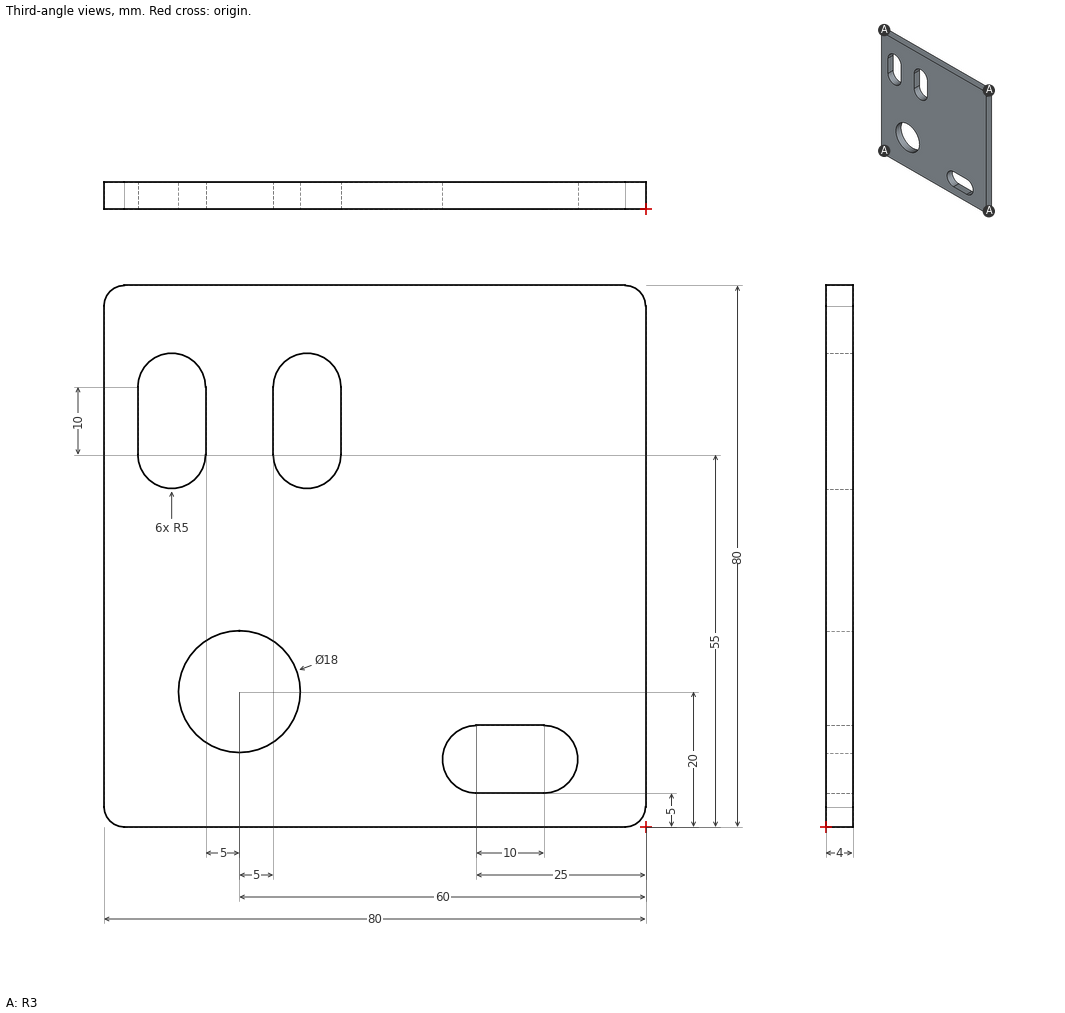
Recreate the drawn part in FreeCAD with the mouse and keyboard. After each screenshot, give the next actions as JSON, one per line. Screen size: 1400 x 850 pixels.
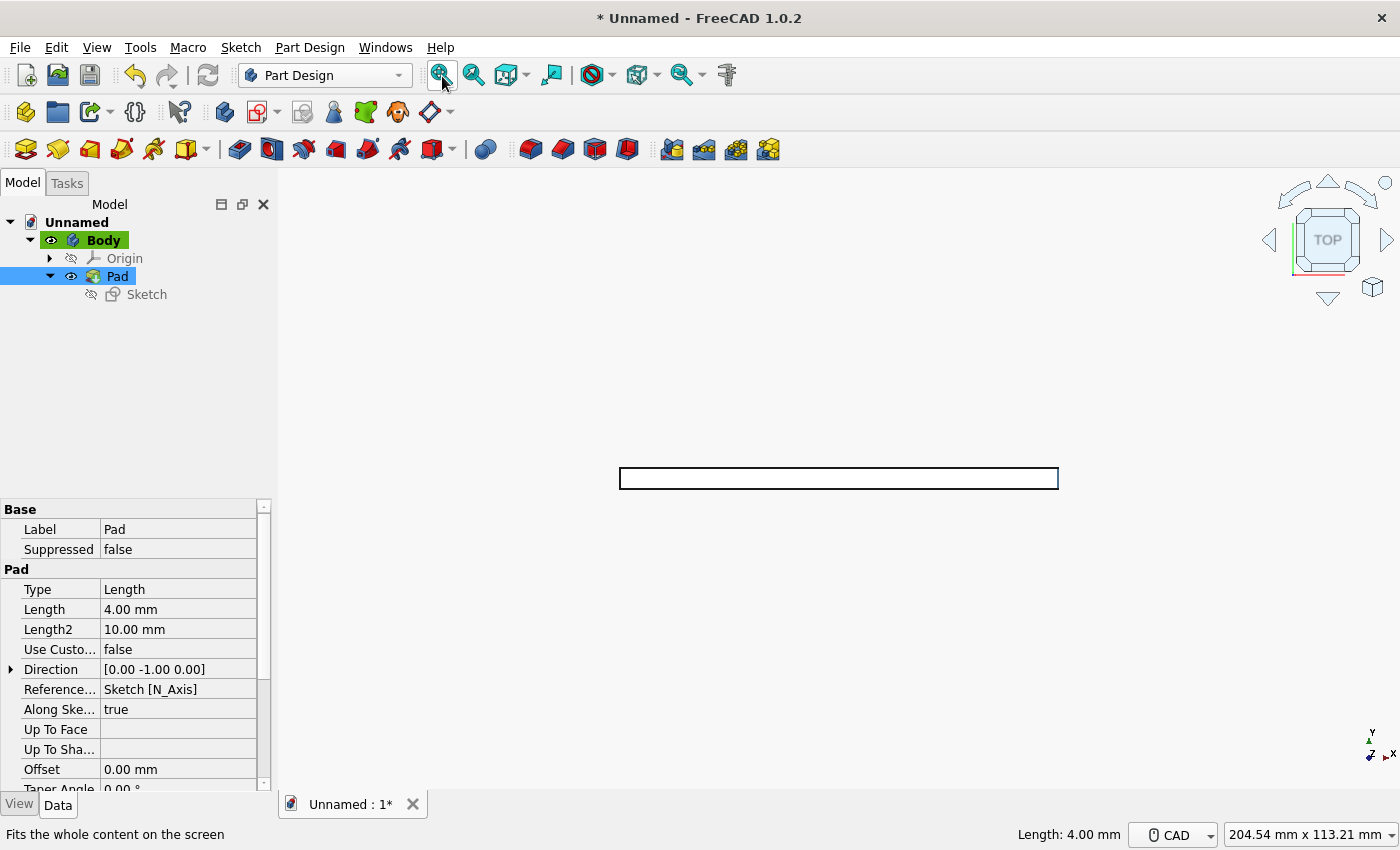
{"action": "left_click", "coordinate": [442, 76]}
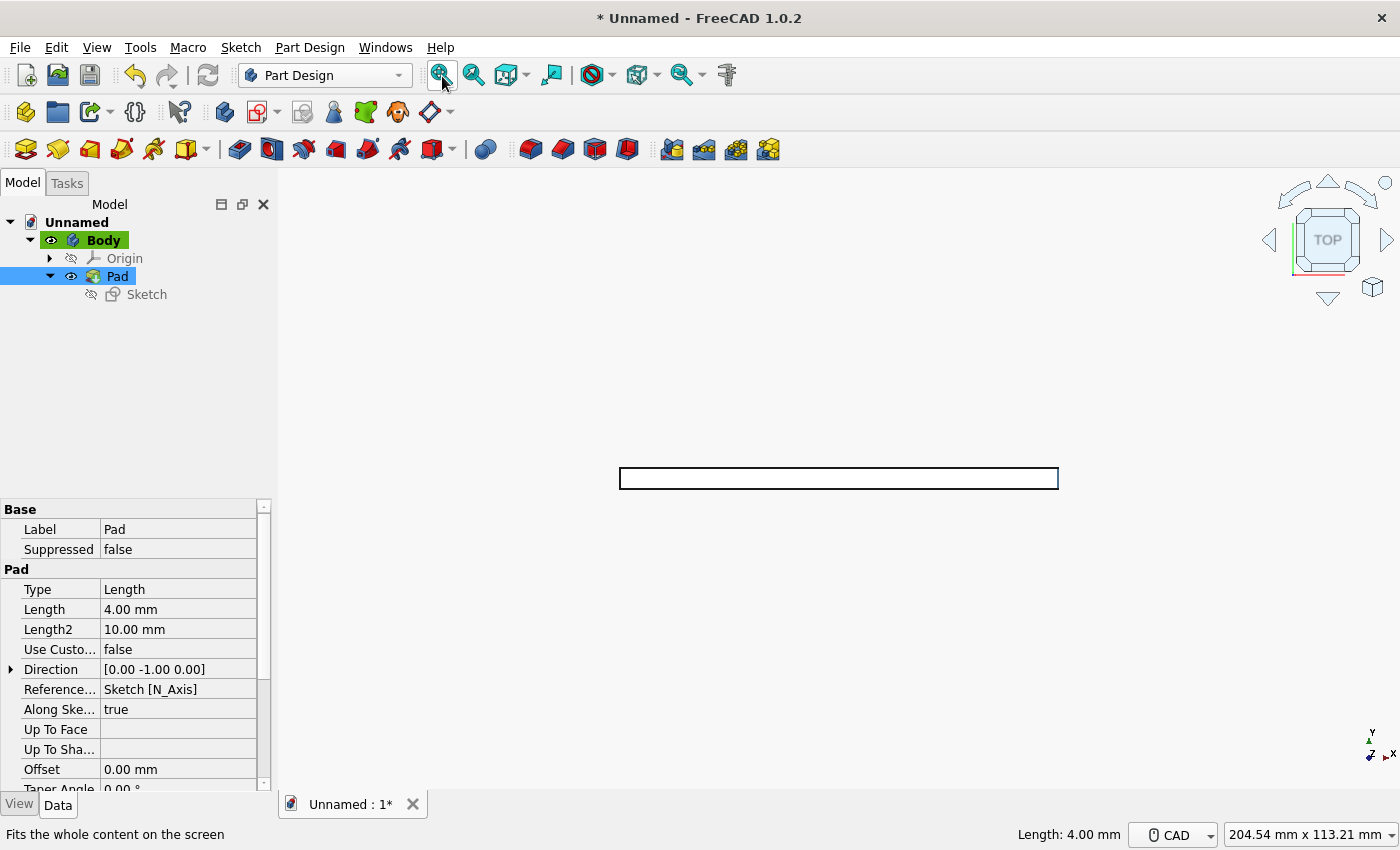
{"action": "left_click", "coordinate": [620, 477], "text": "ctrl"}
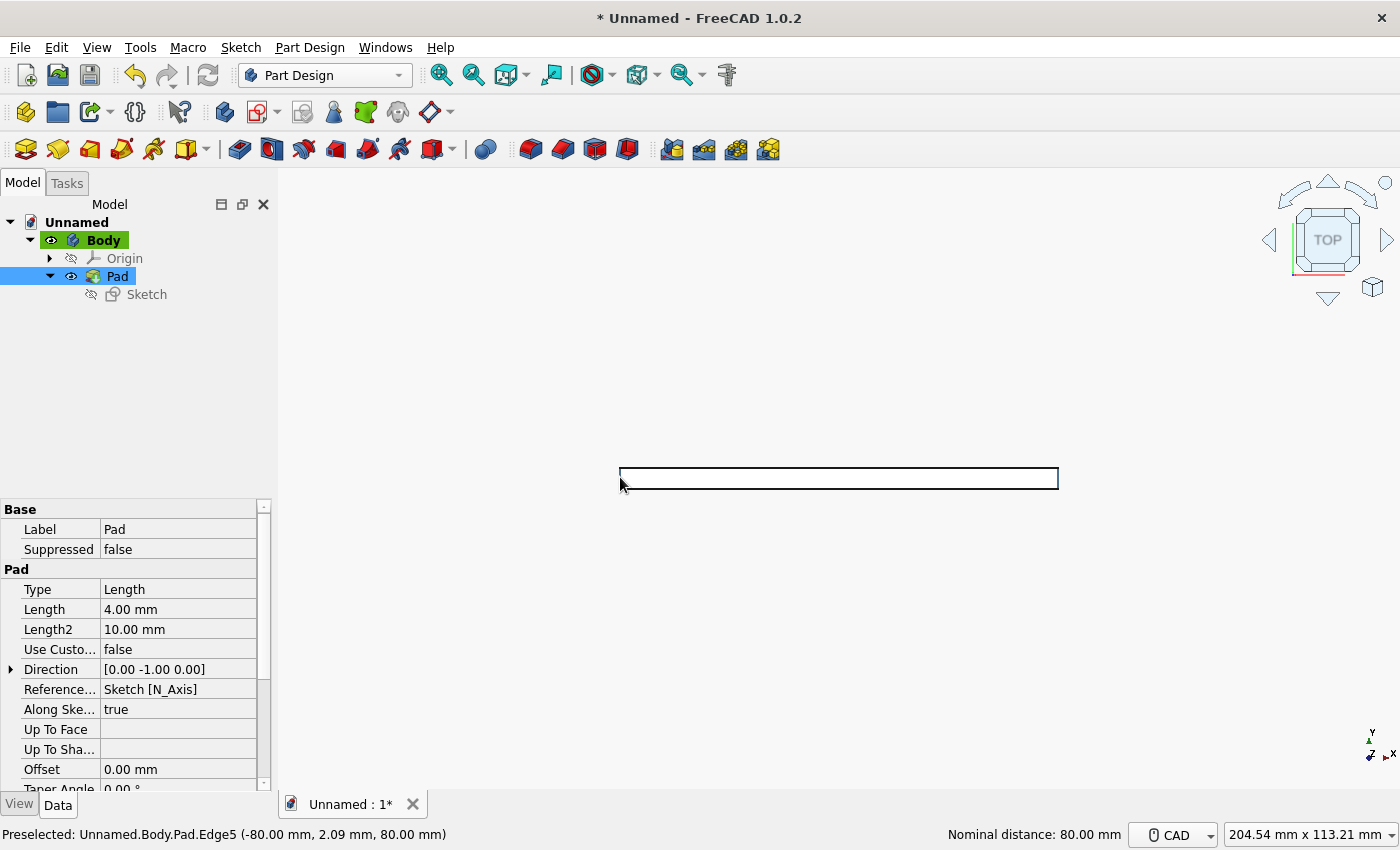
{"action": "scroll", "coordinate": [620, 477], "scroll_direction": "up", "scroll_amount": 4}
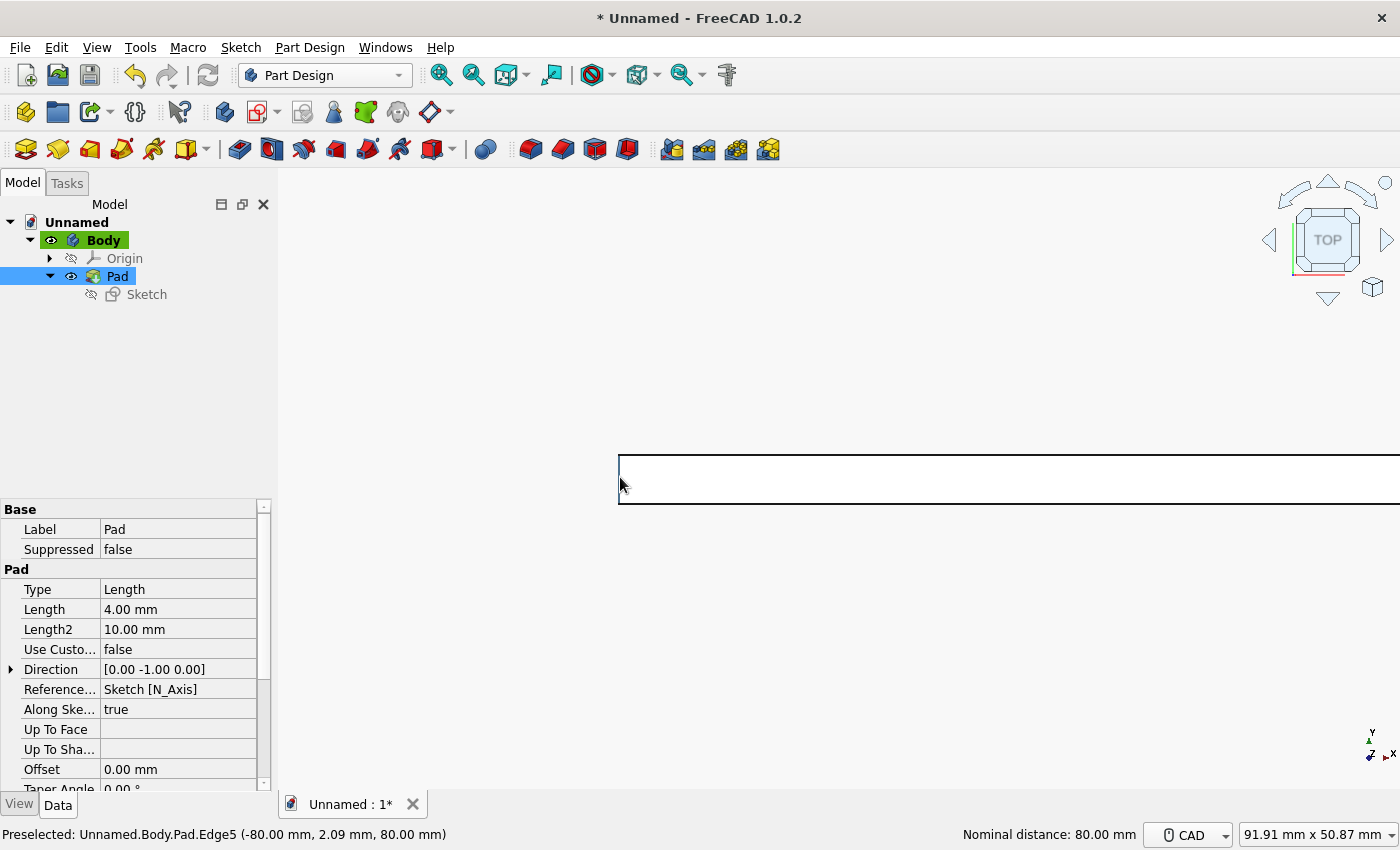
{"action": "left_click", "coordinate": [442, 76]}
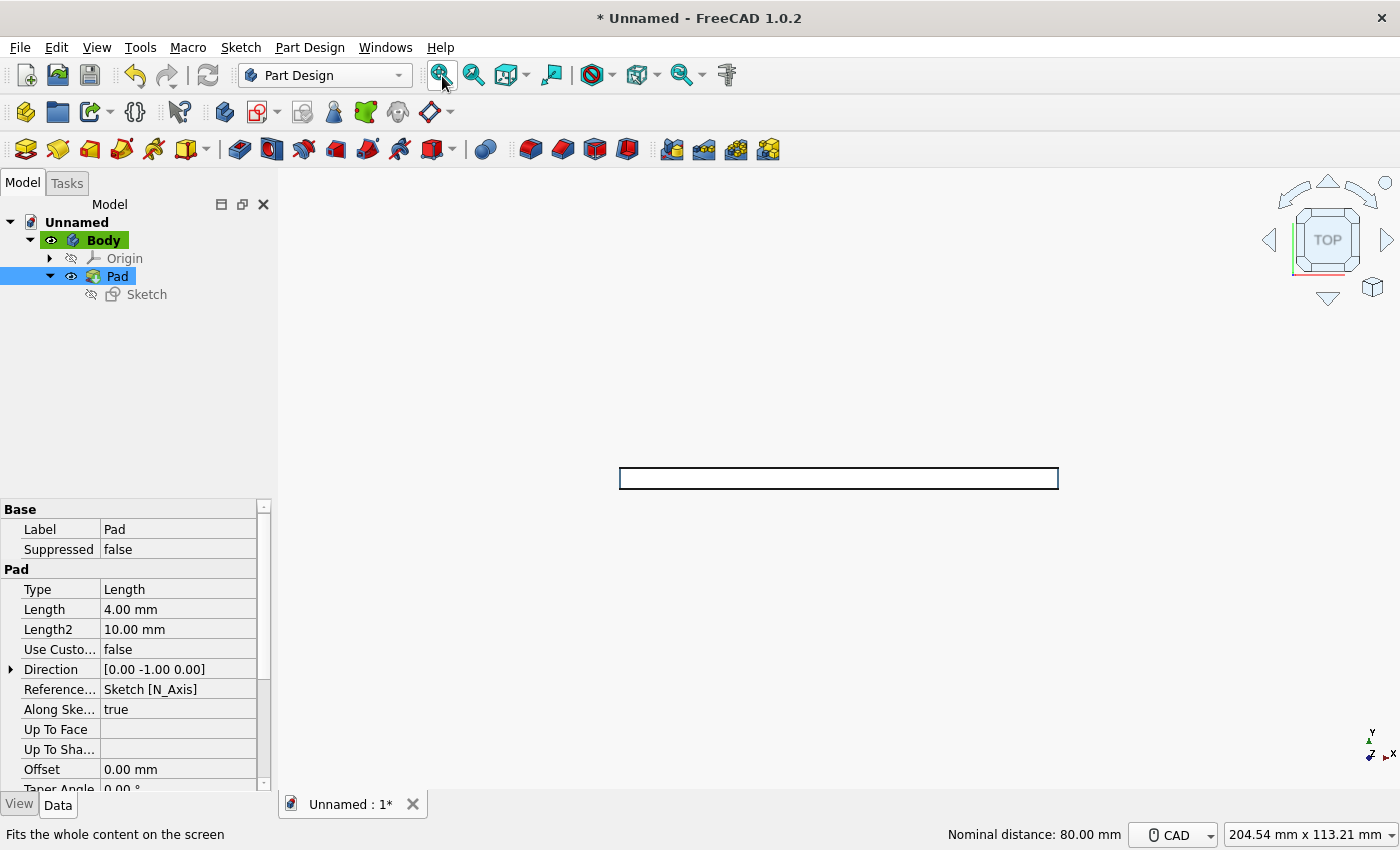
{"action": "key", "text": "1"}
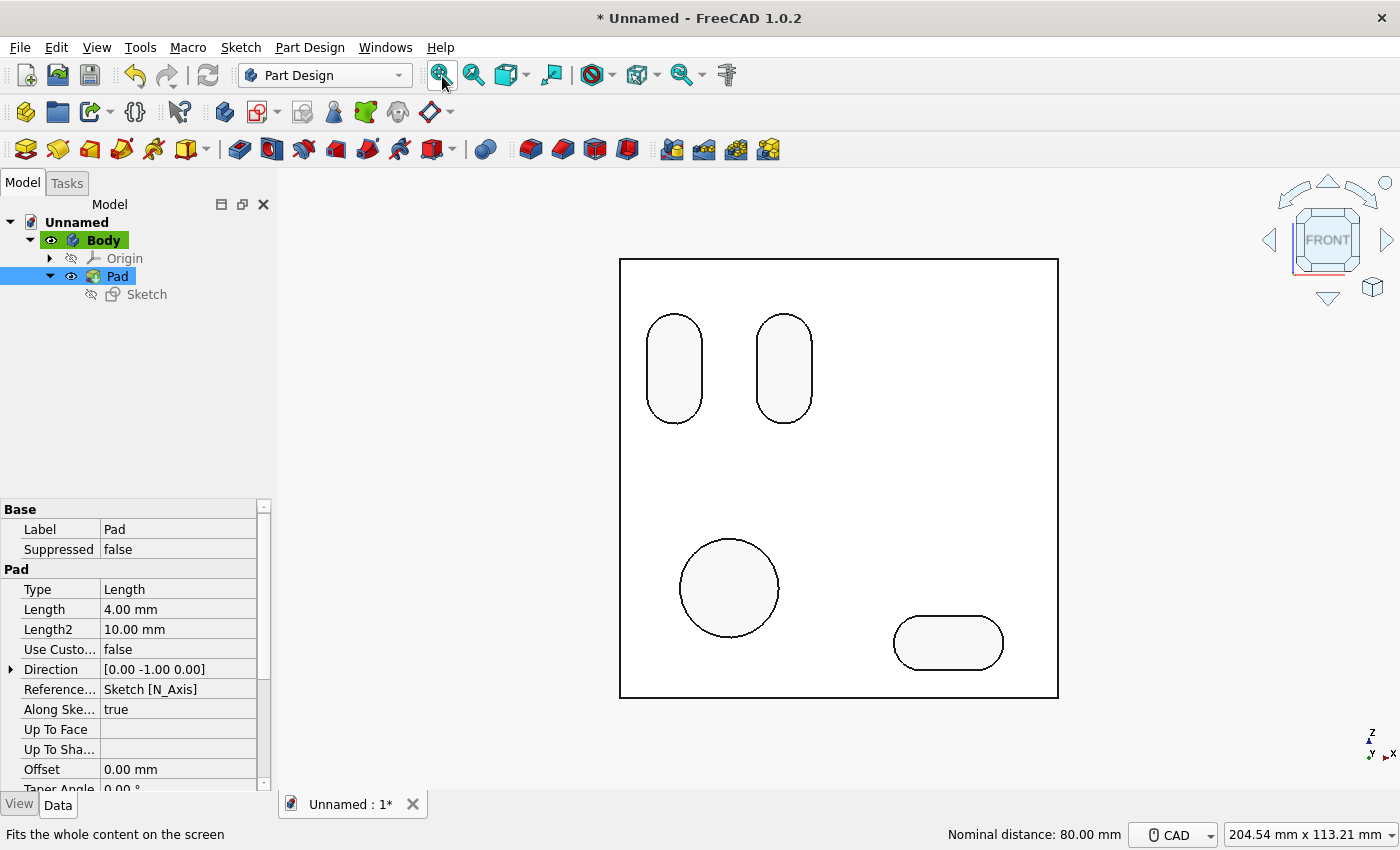
{"action": "scroll", "coordinate": [620, 697], "scroll_direction": "up", "scroll_amount": 4}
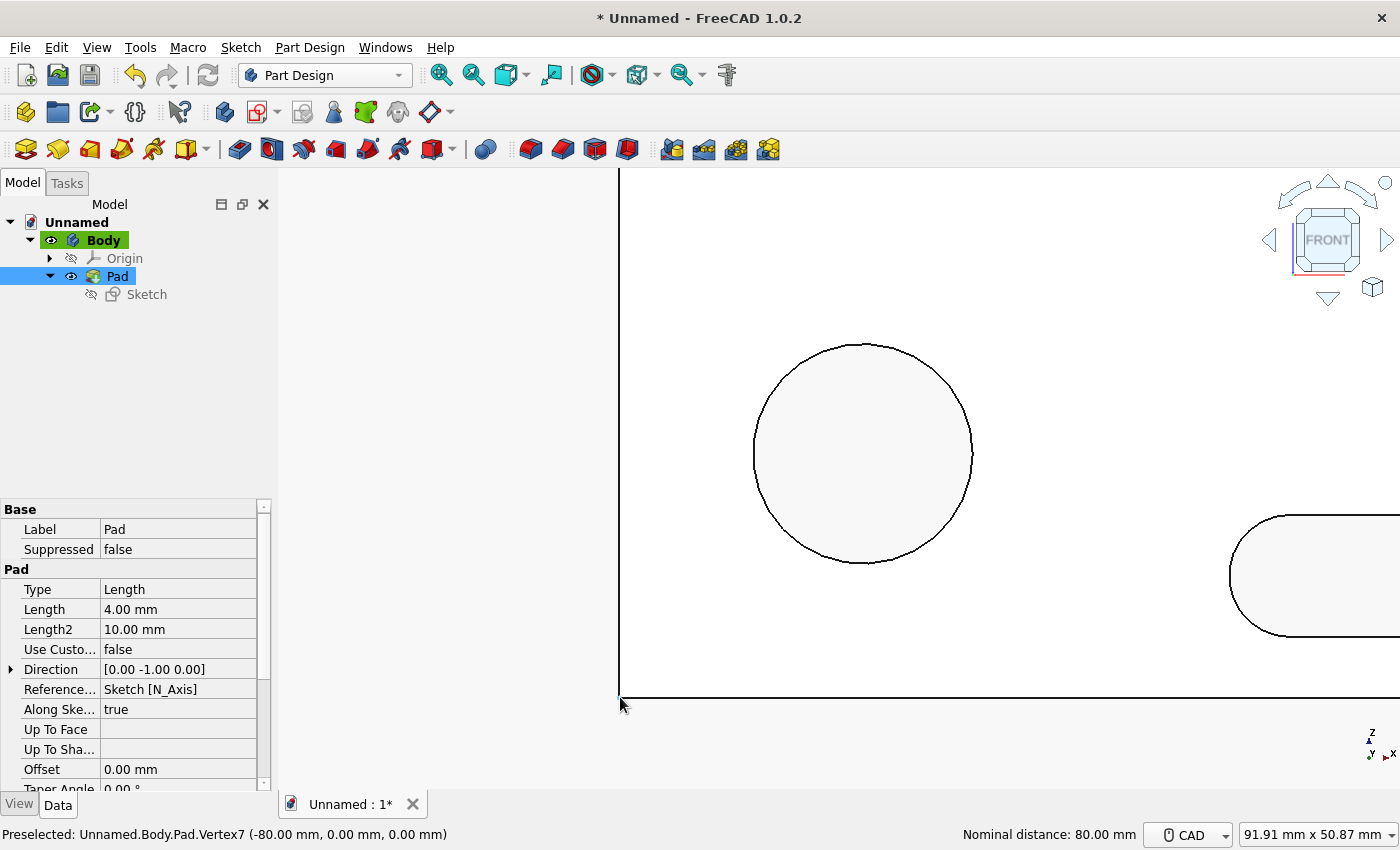
{"action": "left_click", "coordinate": [442, 76]}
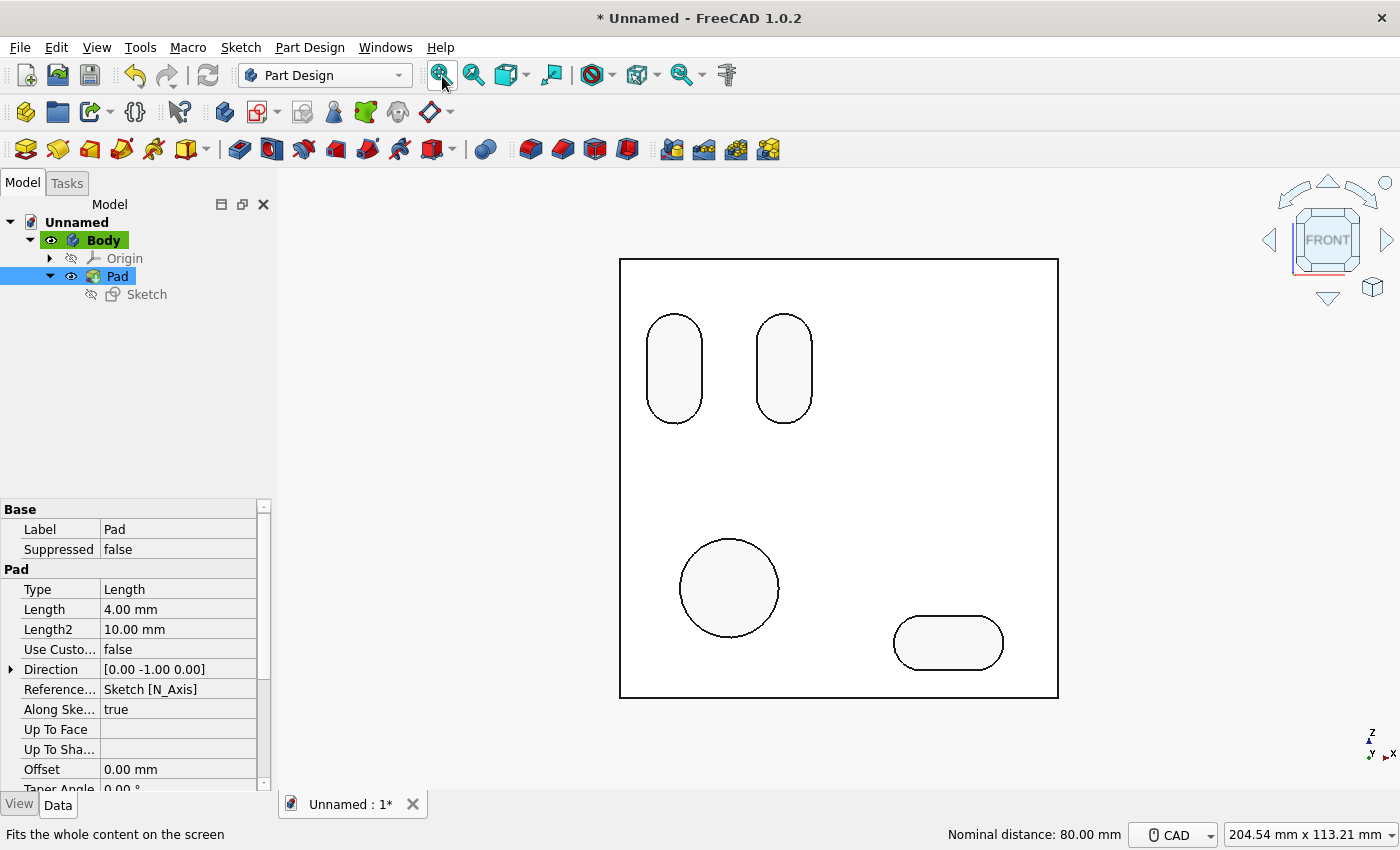
{"action": "key", "text": "3"}